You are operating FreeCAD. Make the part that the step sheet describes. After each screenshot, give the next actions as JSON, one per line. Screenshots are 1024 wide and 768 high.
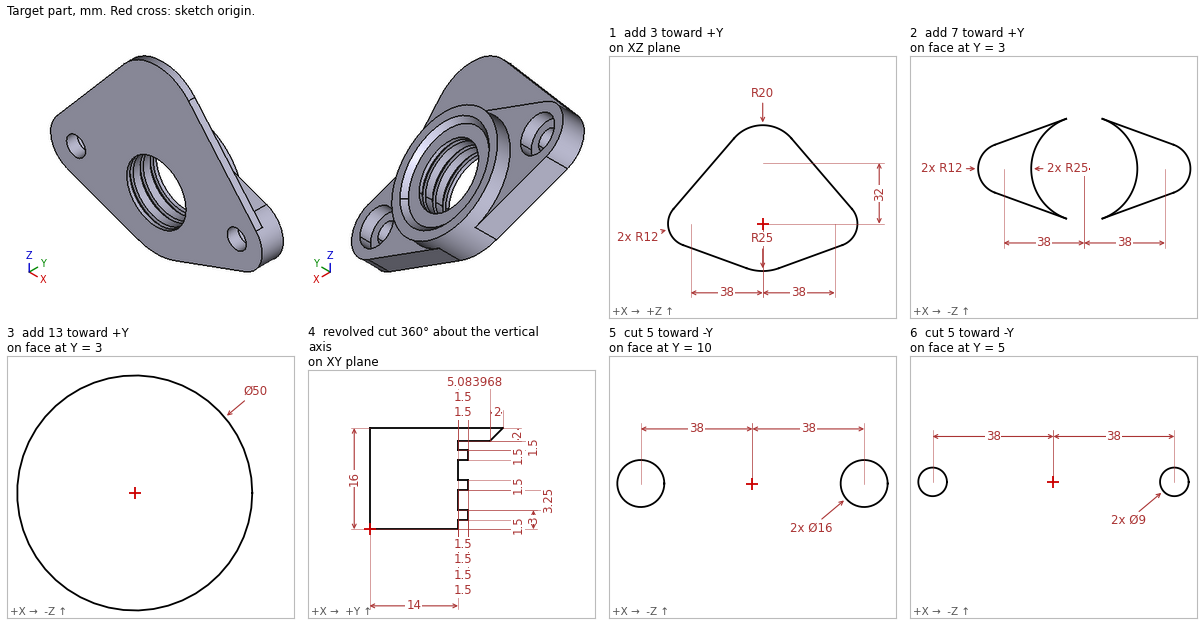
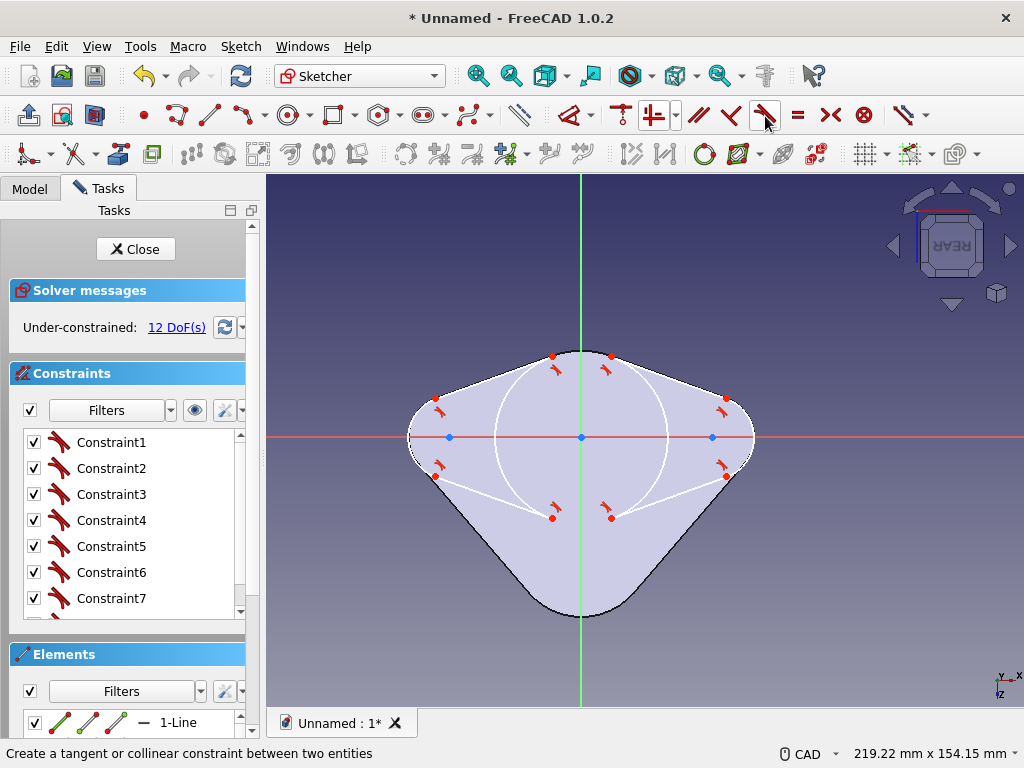
{"action": "left_click", "coordinate": [505, 397]}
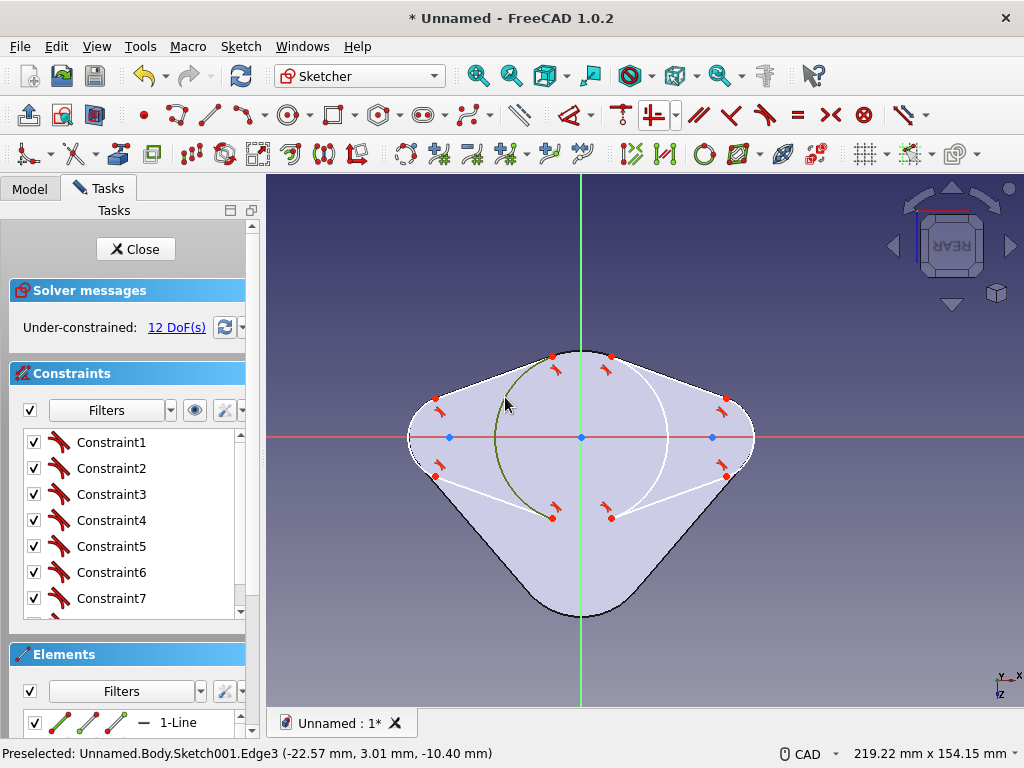
{"action": "left_click", "coordinate": [658, 478]}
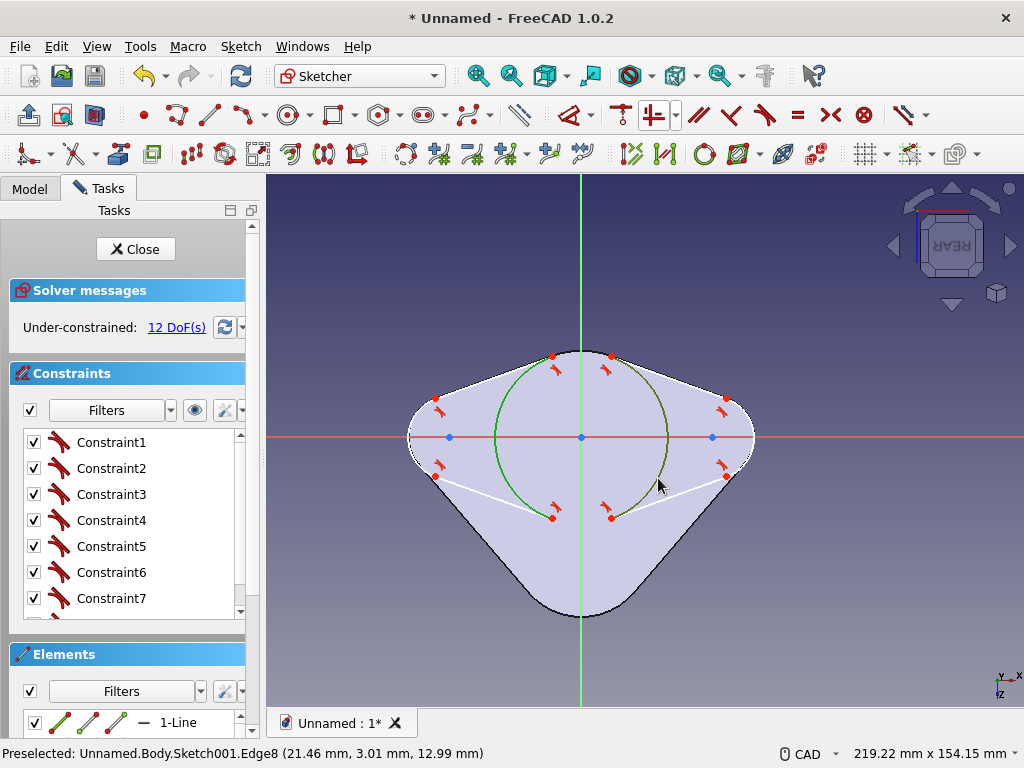
{"action": "left_click", "coordinate": [621, 116]}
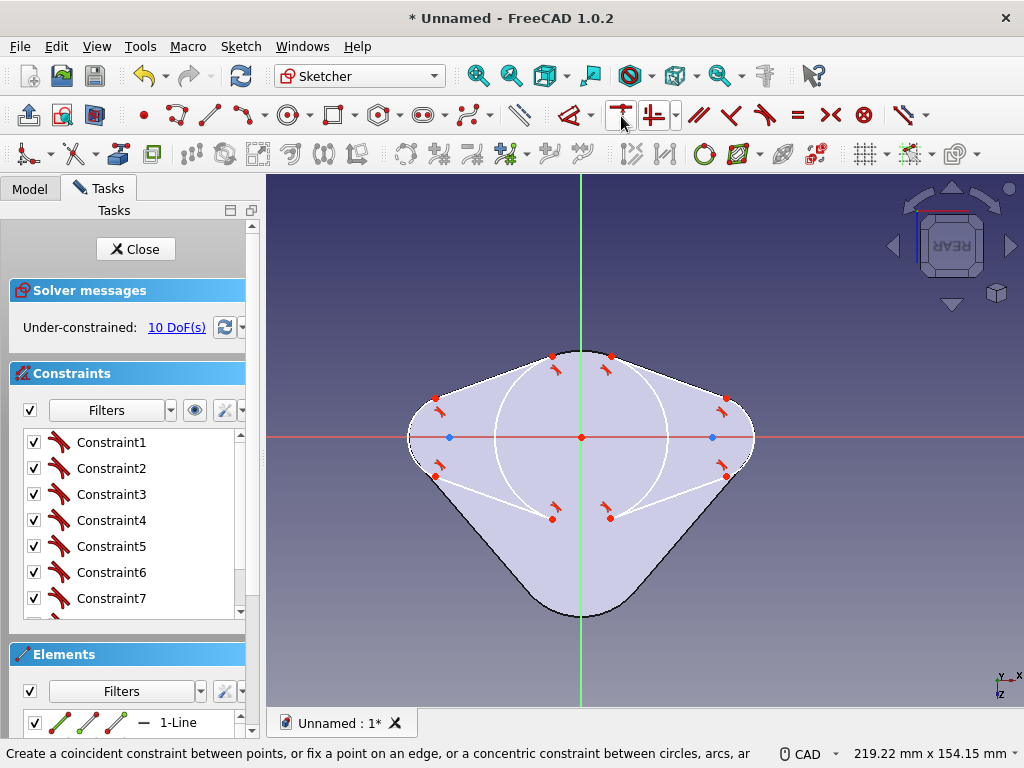
{"action": "left_click_drag", "start_coordinate": [571, 427], "coordinate": [592, 448]}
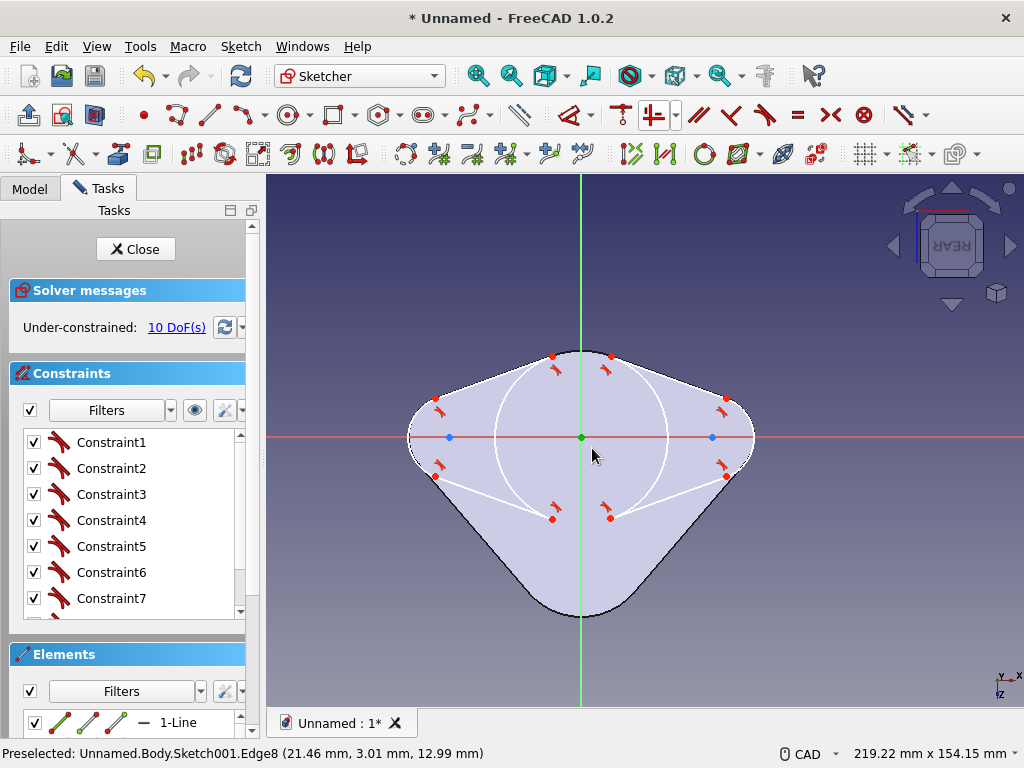
{"action": "left_click", "coordinate": [621, 116]}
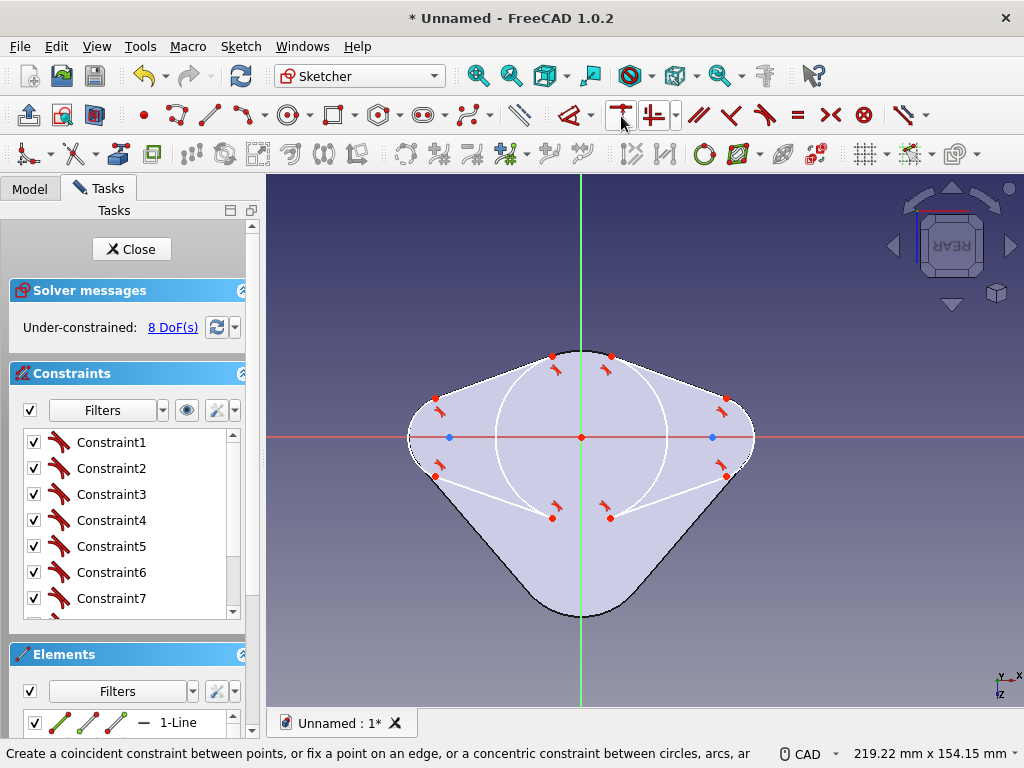
{"action": "left_click", "coordinate": [413, 419]}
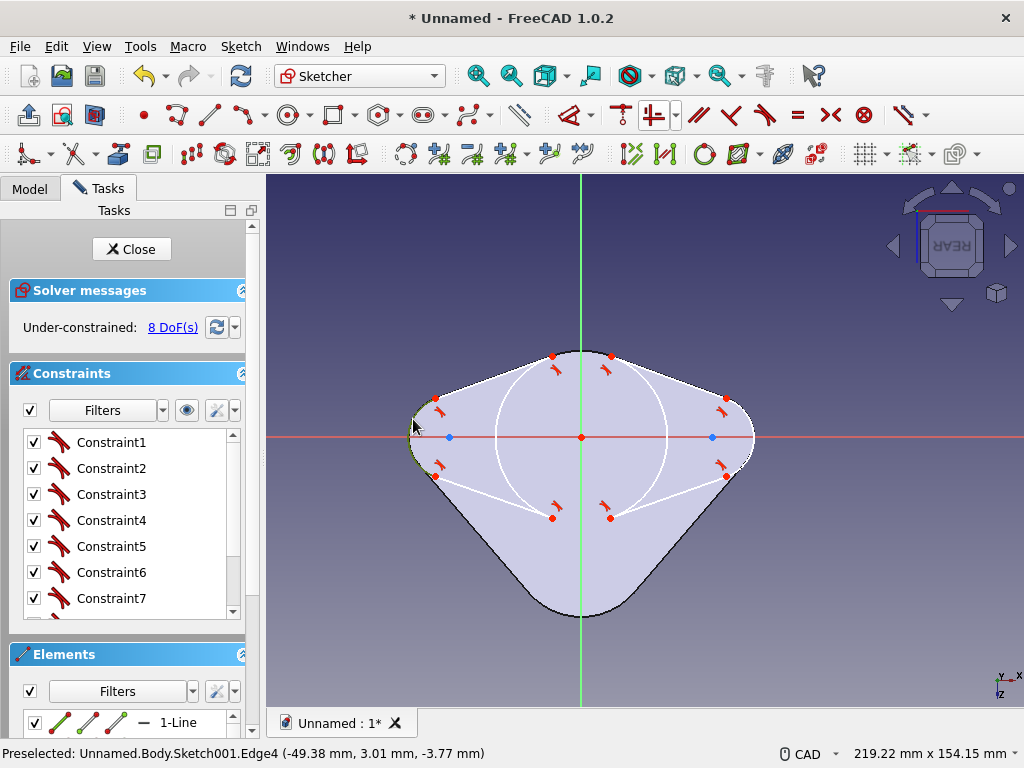
{"action": "left_click", "coordinate": [749, 458]}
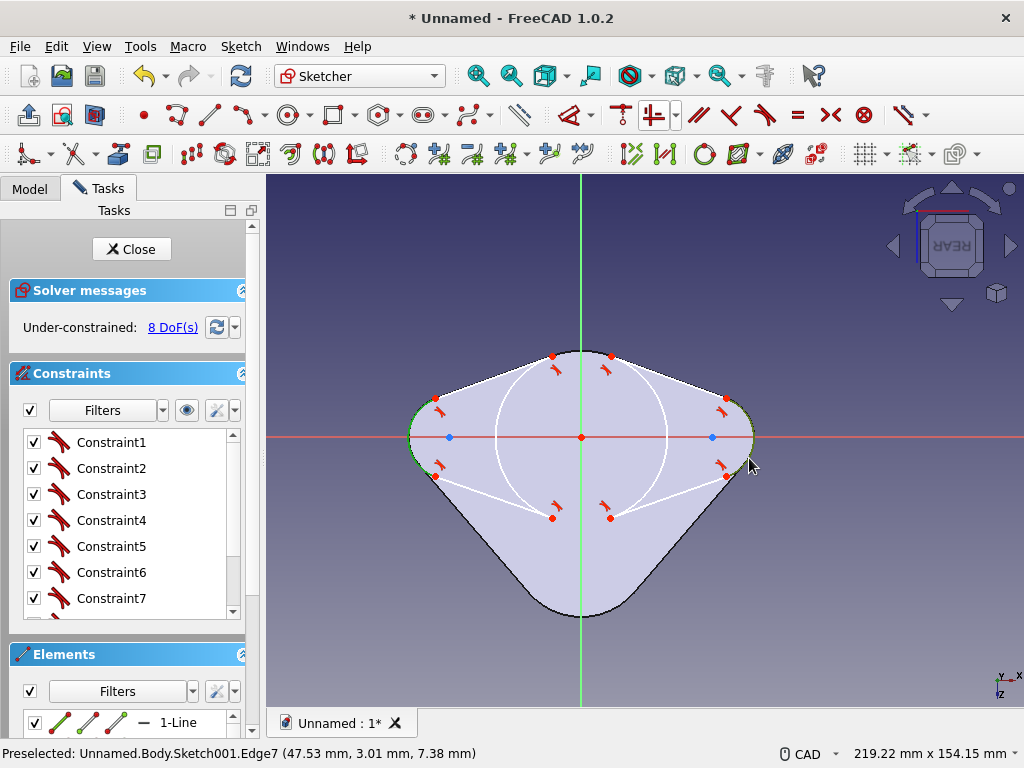
{"action": "left_click", "coordinate": [798, 116]}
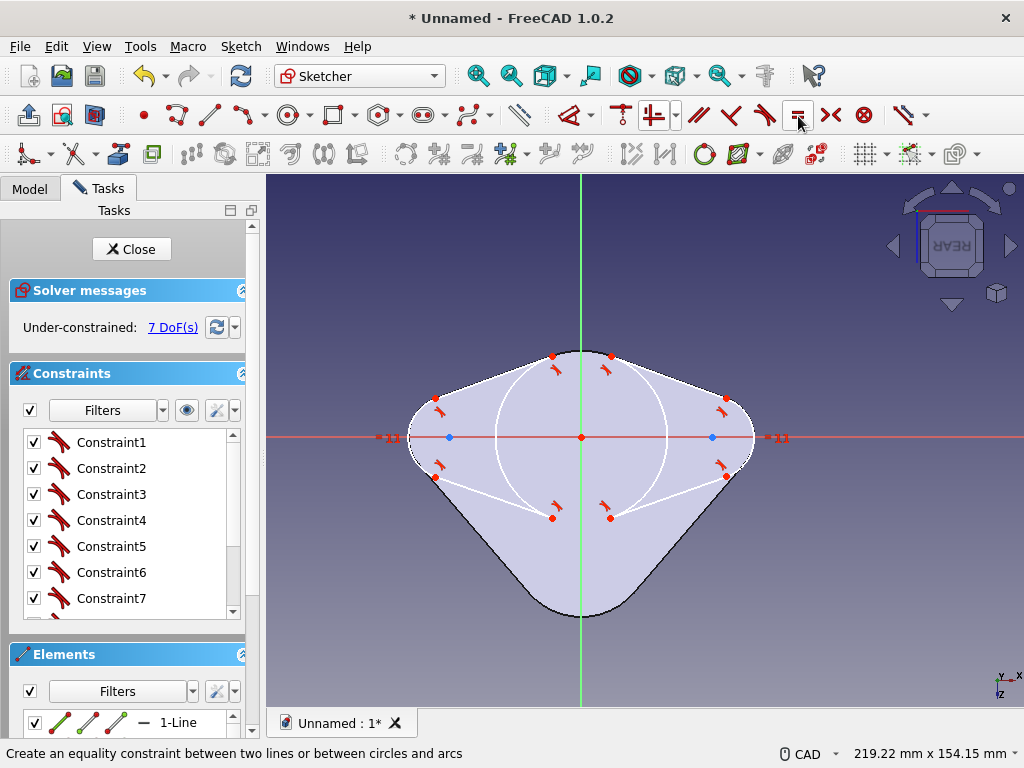
{"action": "left_click", "coordinate": [505, 397]}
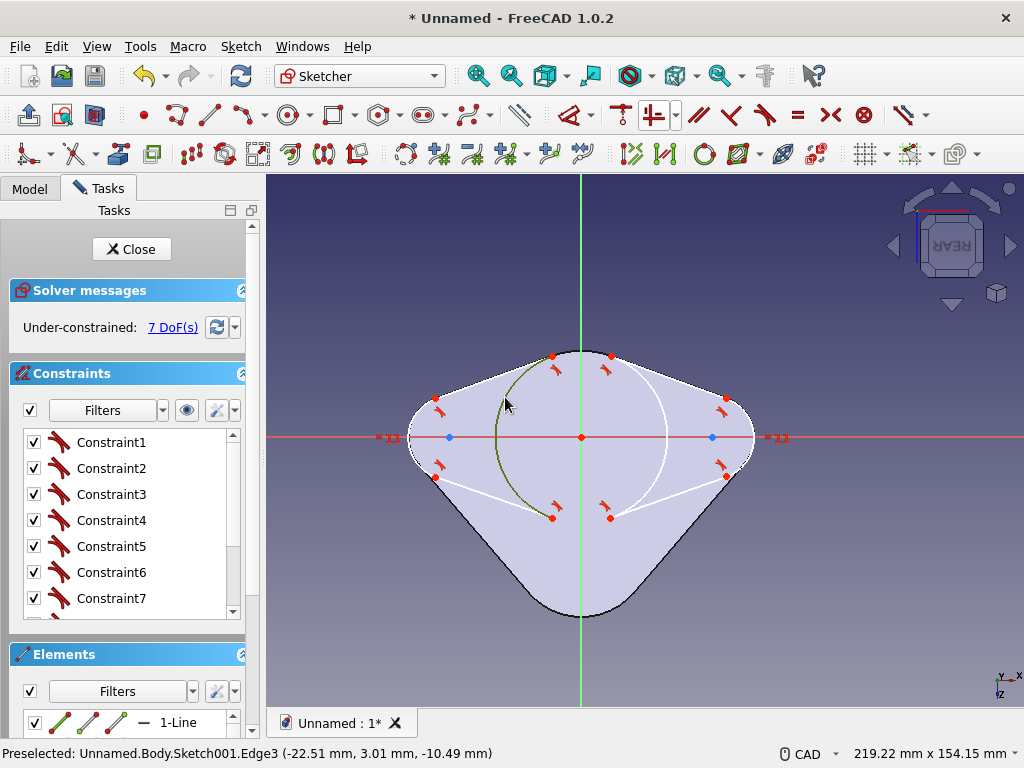
{"action": "left_click", "coordinate": [657, 478]}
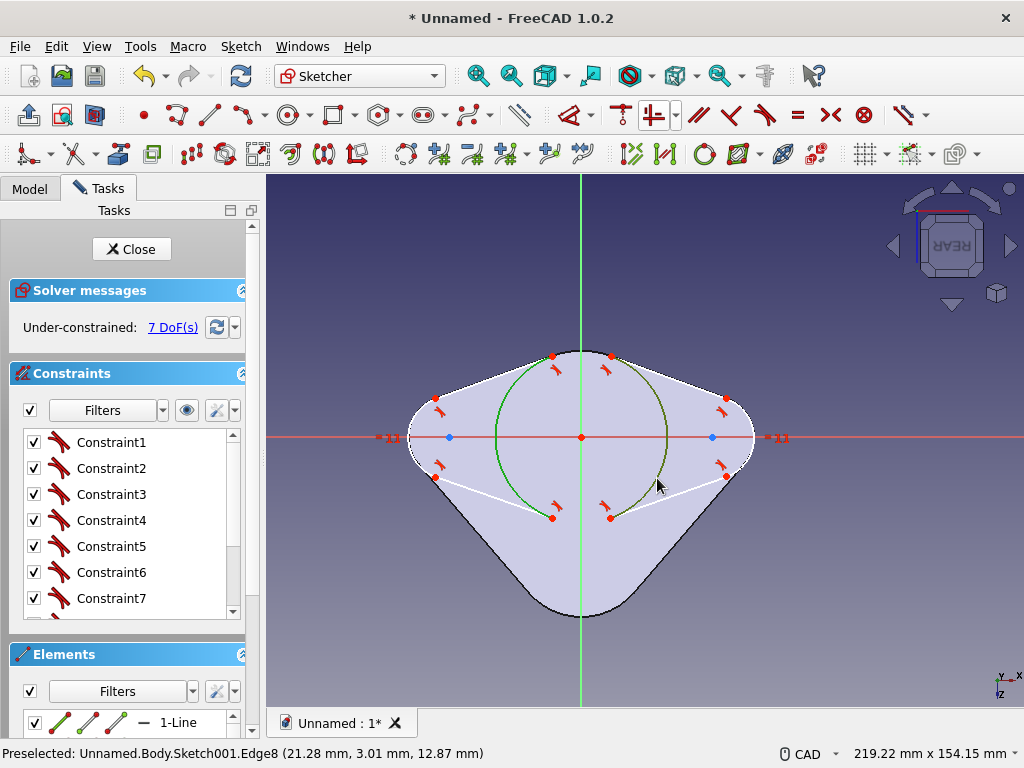
{"action": "left_click", "coordinate": [798, 116]}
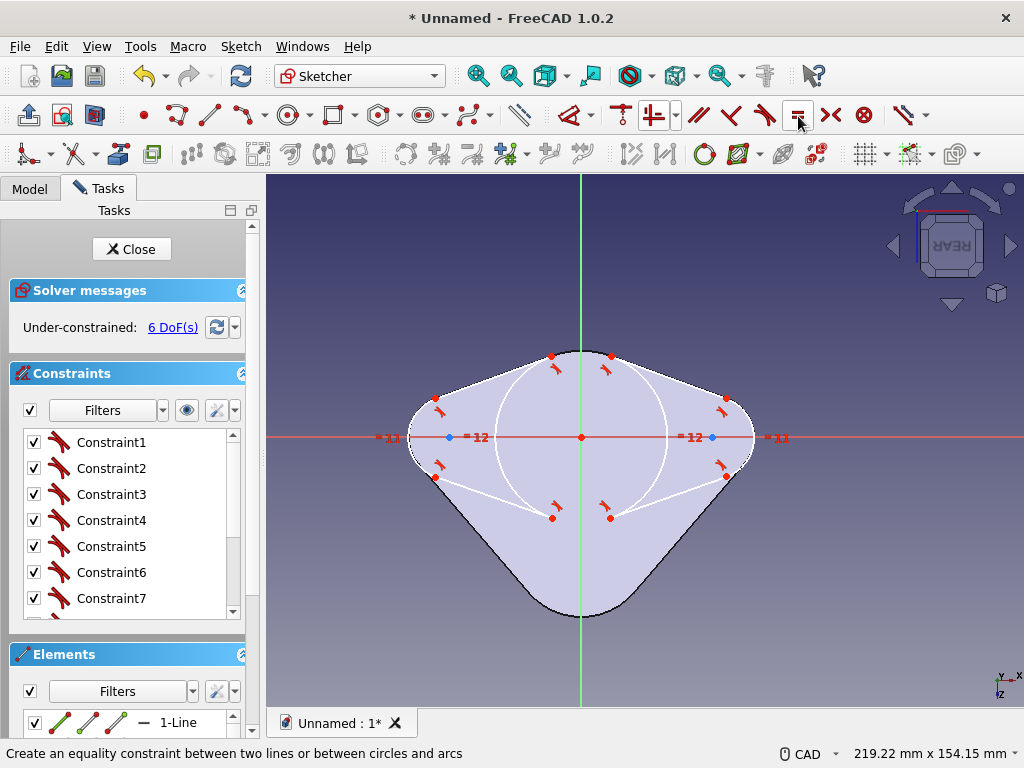
{"action": "left_click", "coordinate": [450, 438]}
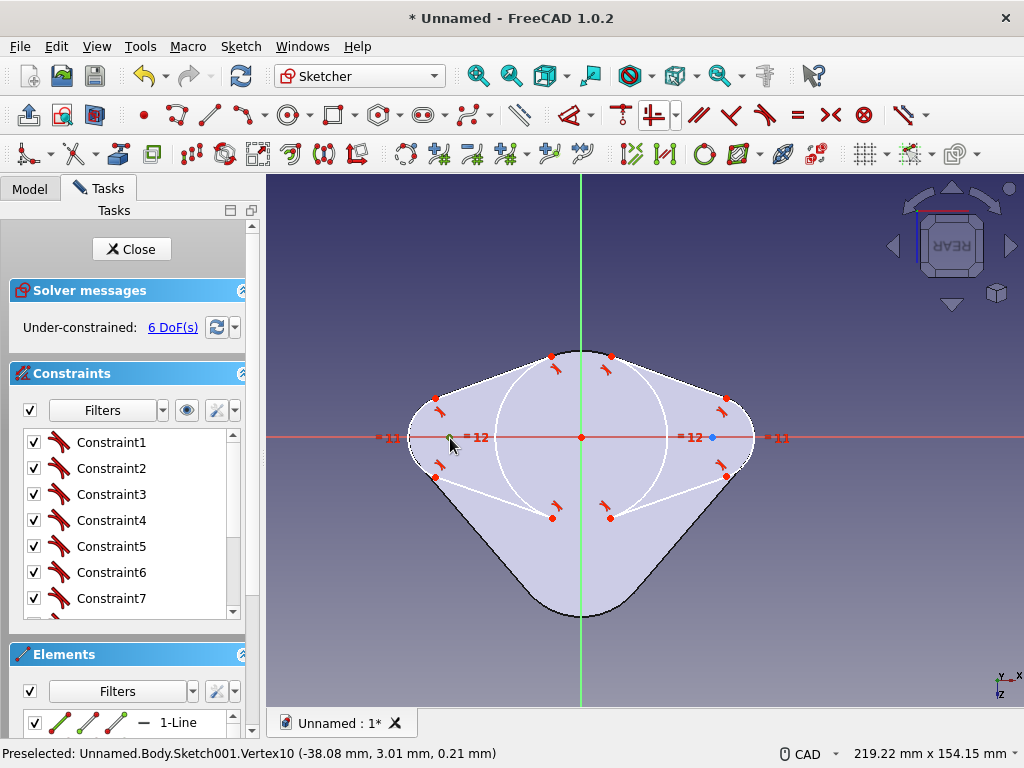
{"action": "left_click", "coordinate": [334, 437]}